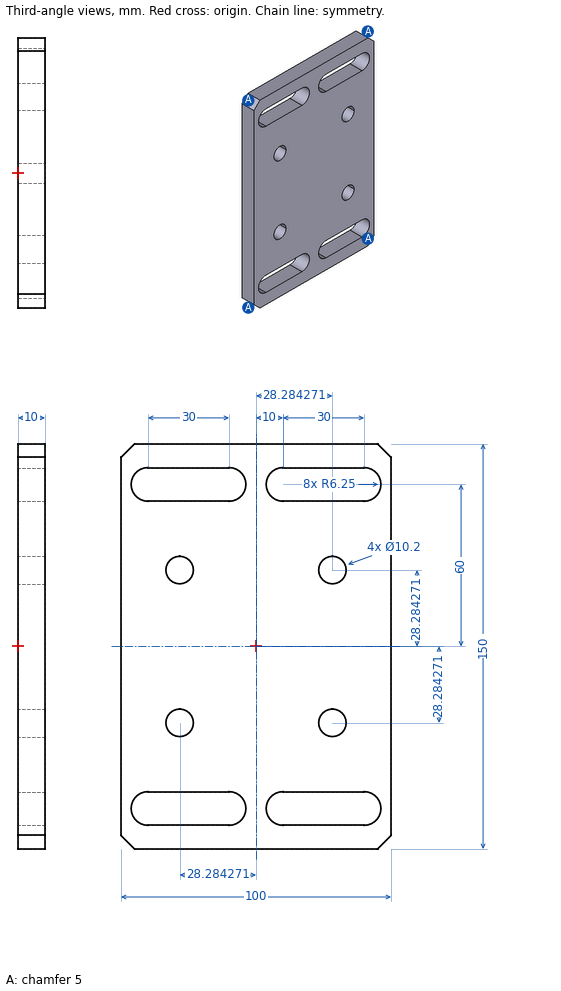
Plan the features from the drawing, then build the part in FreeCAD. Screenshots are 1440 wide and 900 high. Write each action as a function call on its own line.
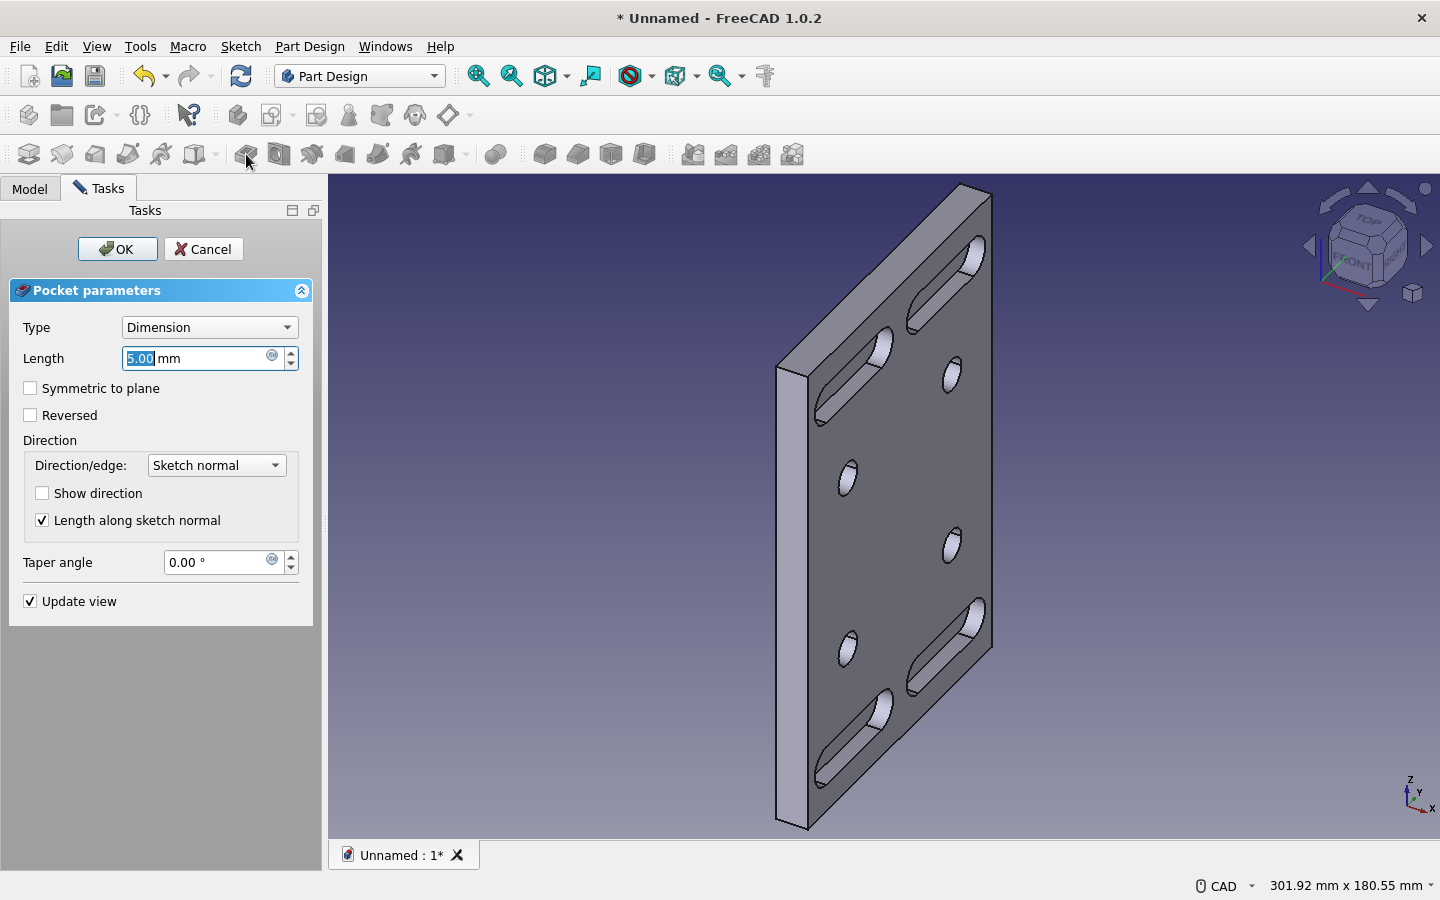
click(210, 328)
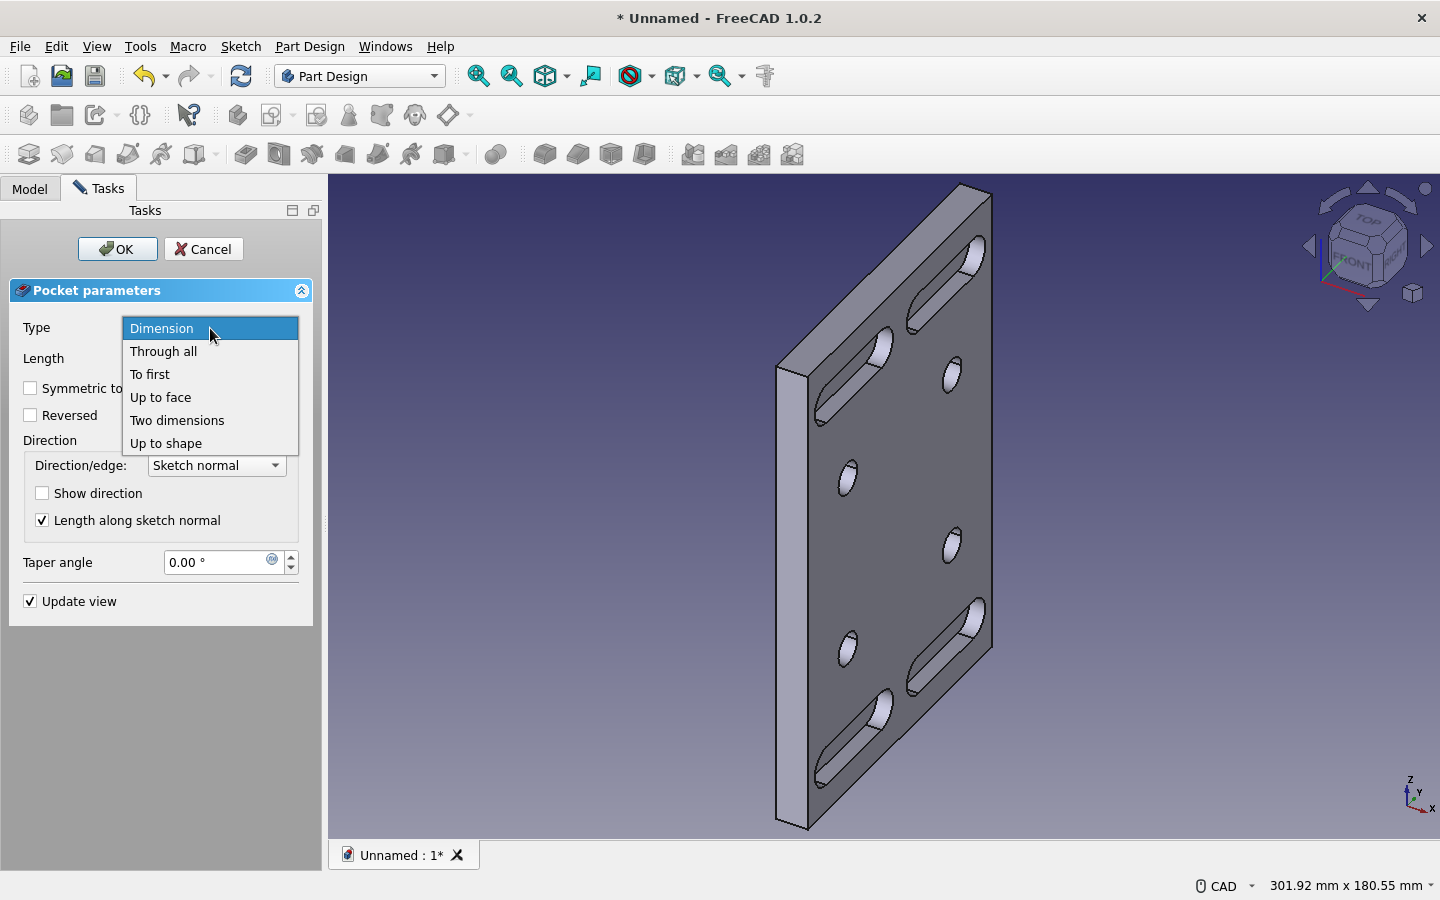
click(208, 352)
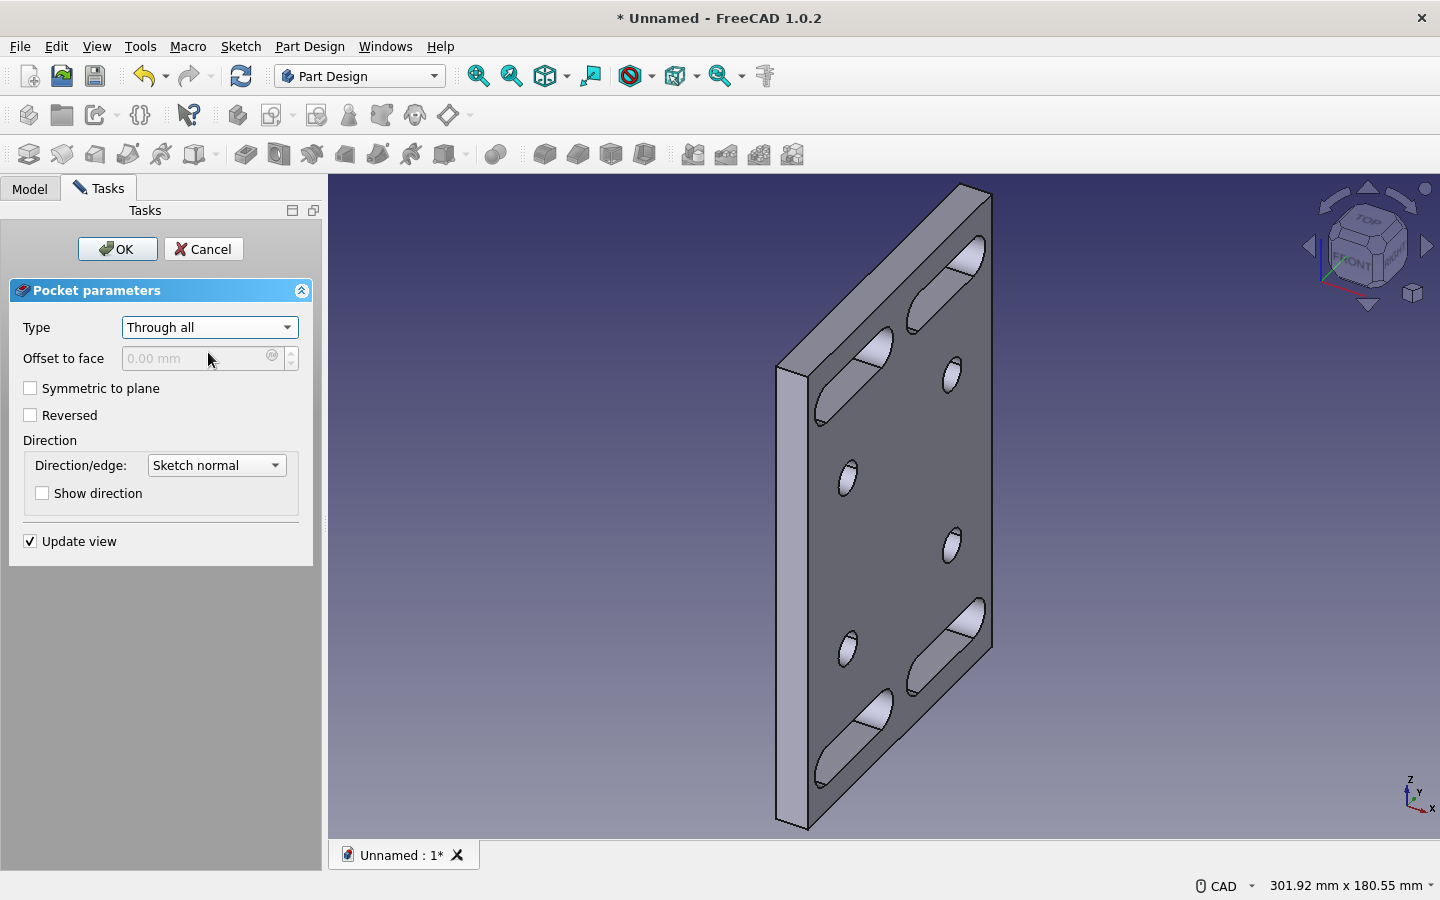
click(118, 249)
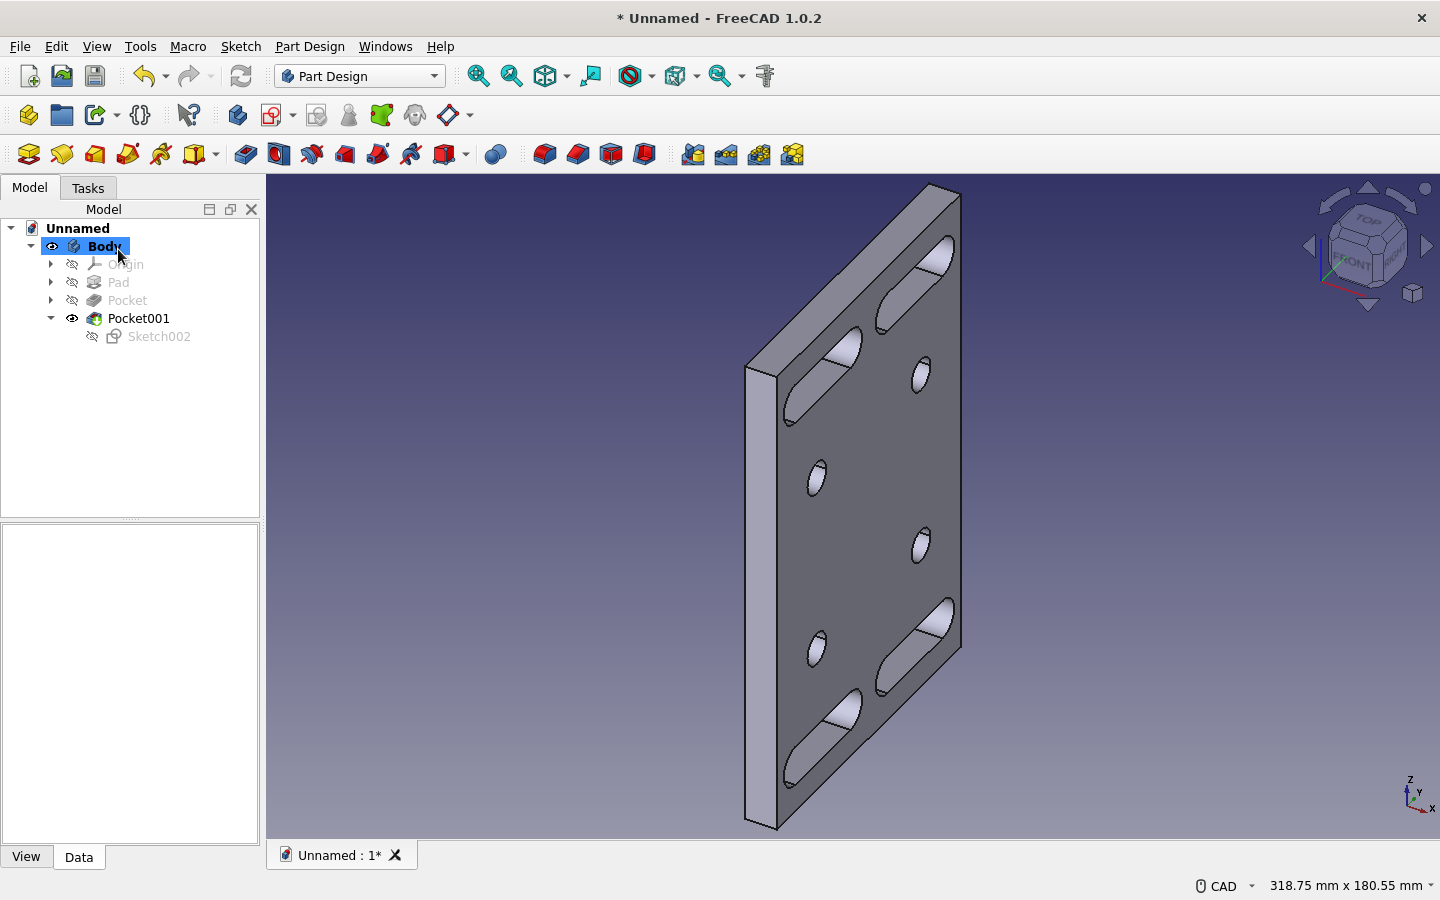
click(761, 371)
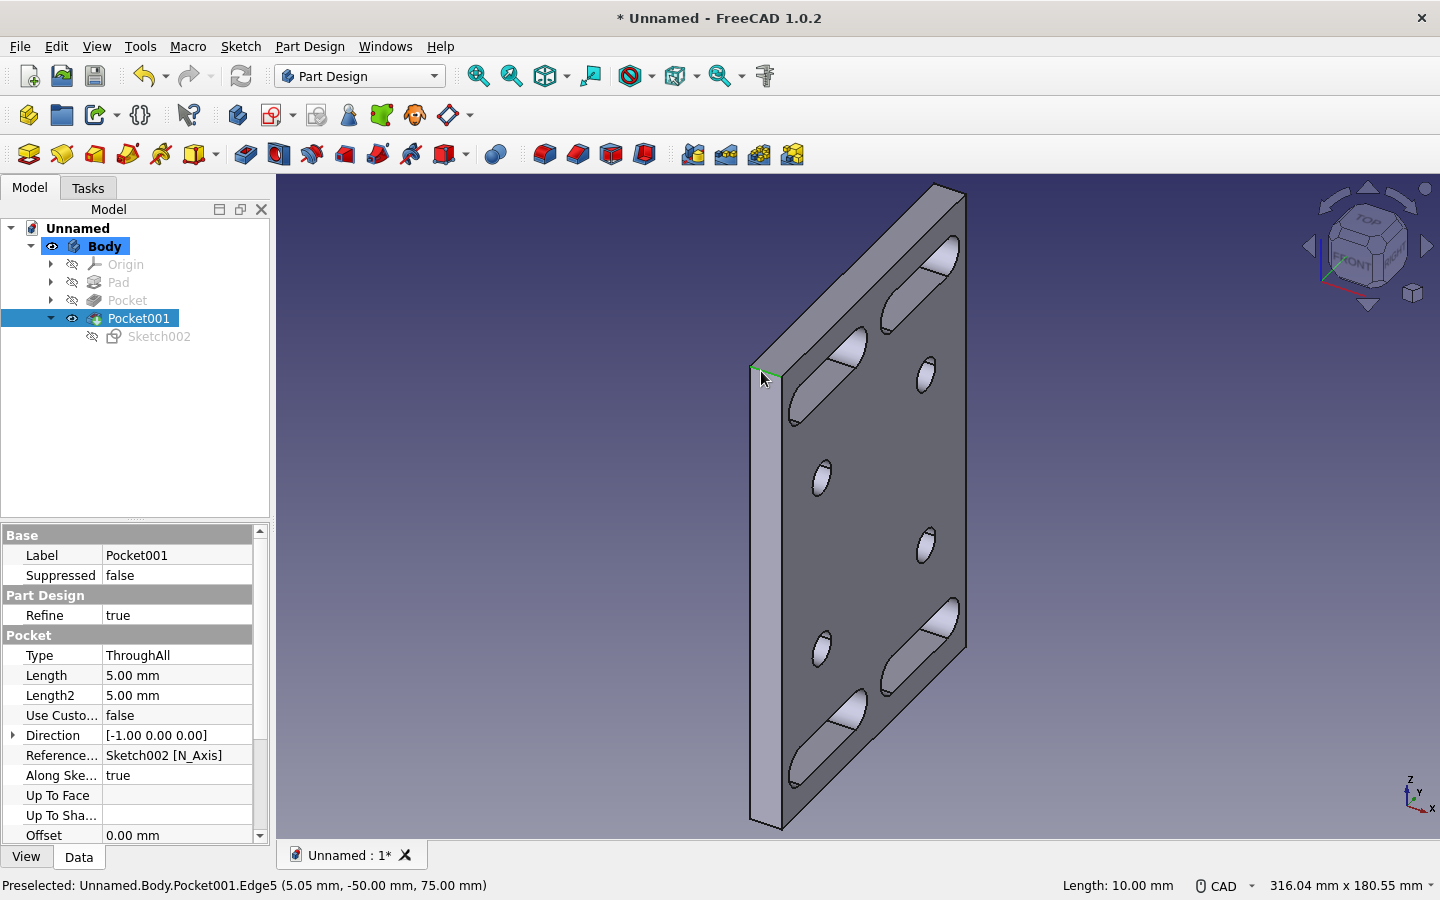
key(0)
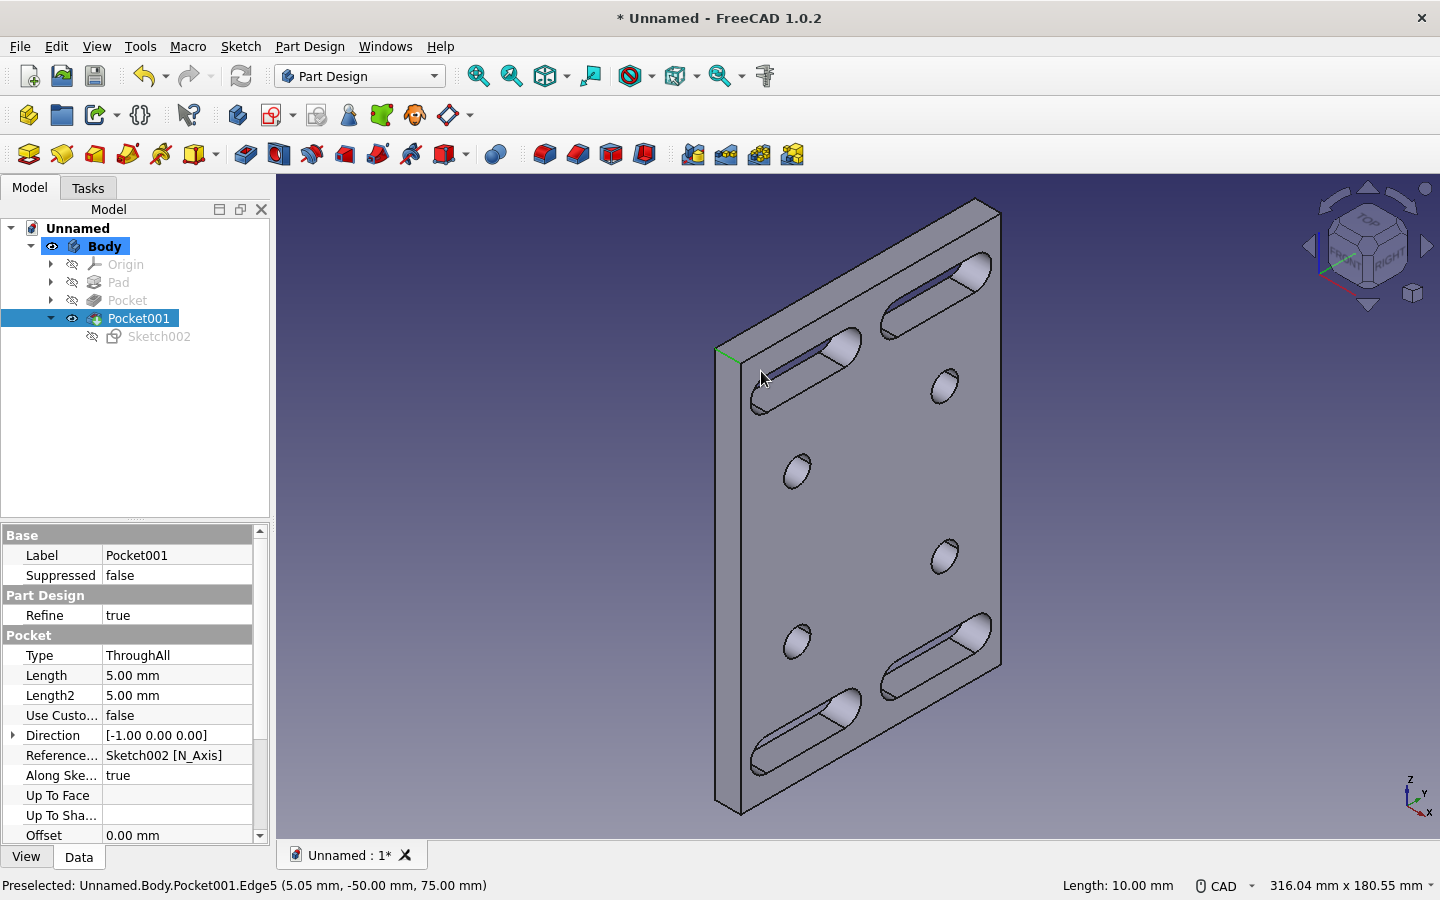
key(2)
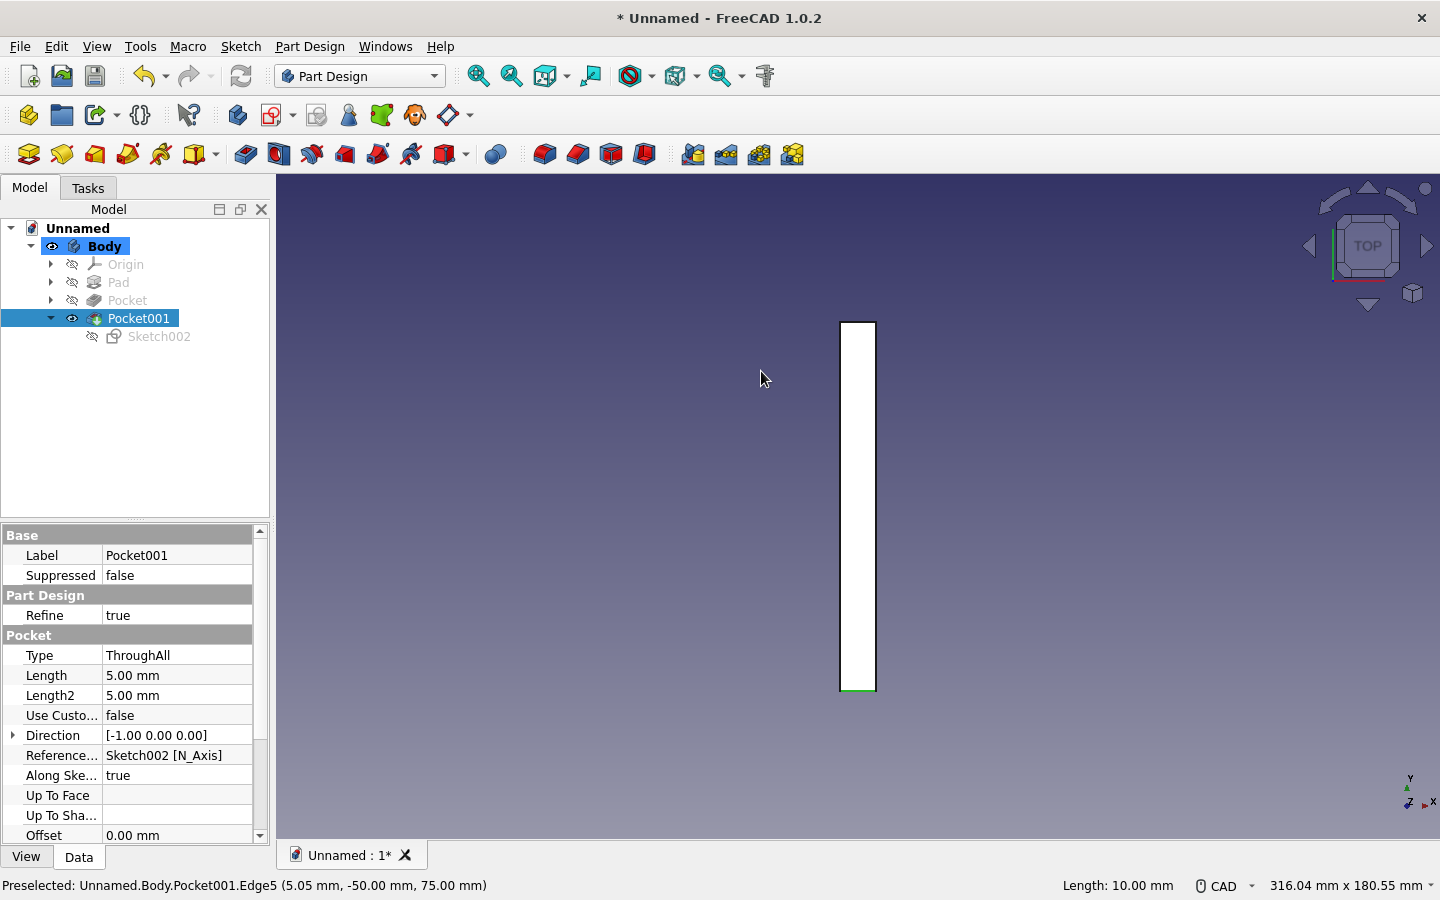
click(858, 321, ctrl)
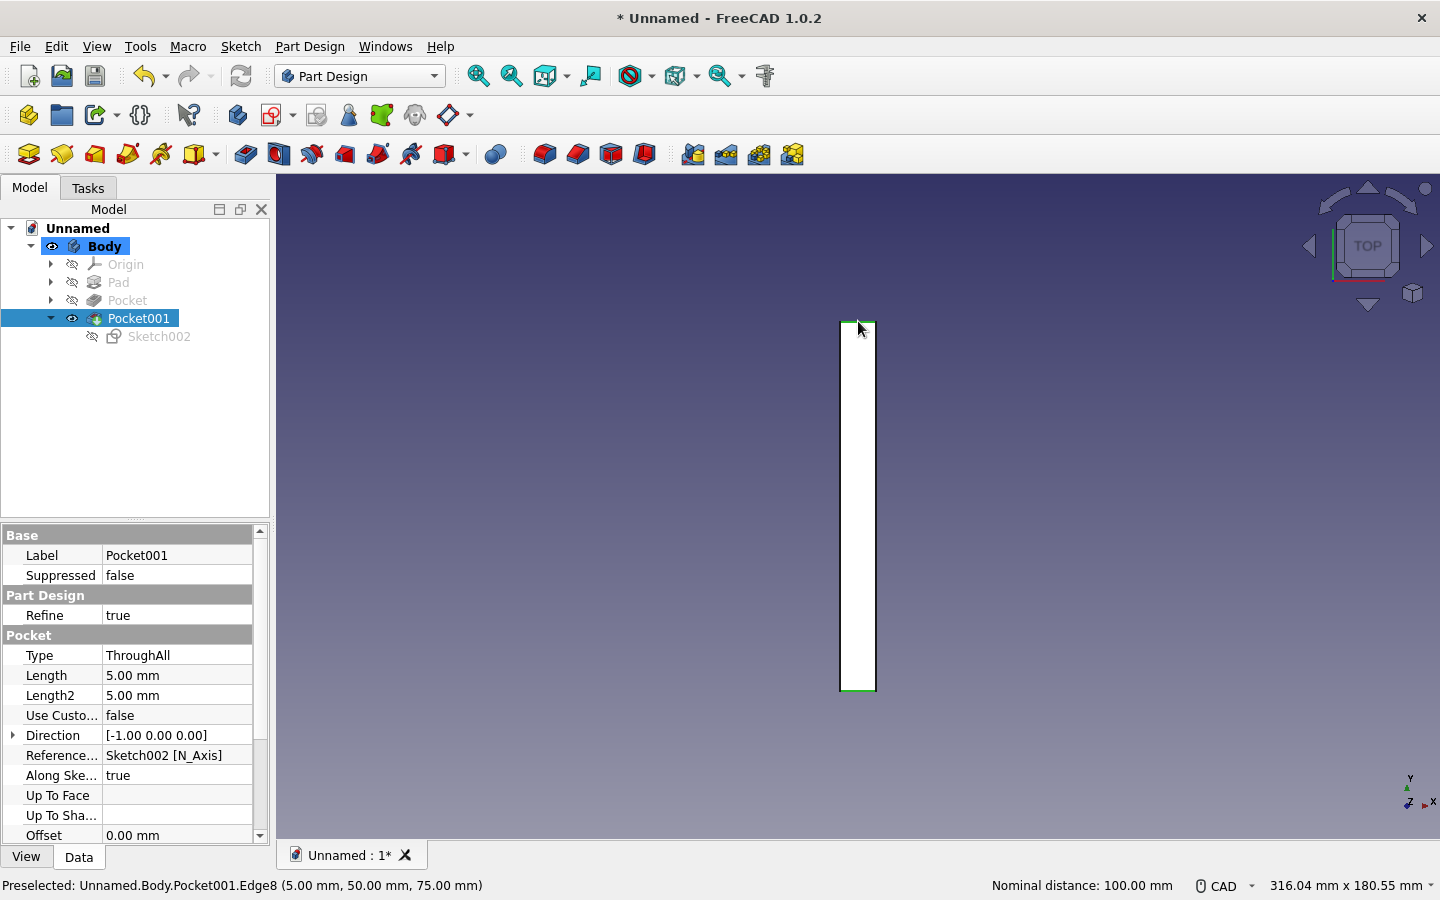
key(1)